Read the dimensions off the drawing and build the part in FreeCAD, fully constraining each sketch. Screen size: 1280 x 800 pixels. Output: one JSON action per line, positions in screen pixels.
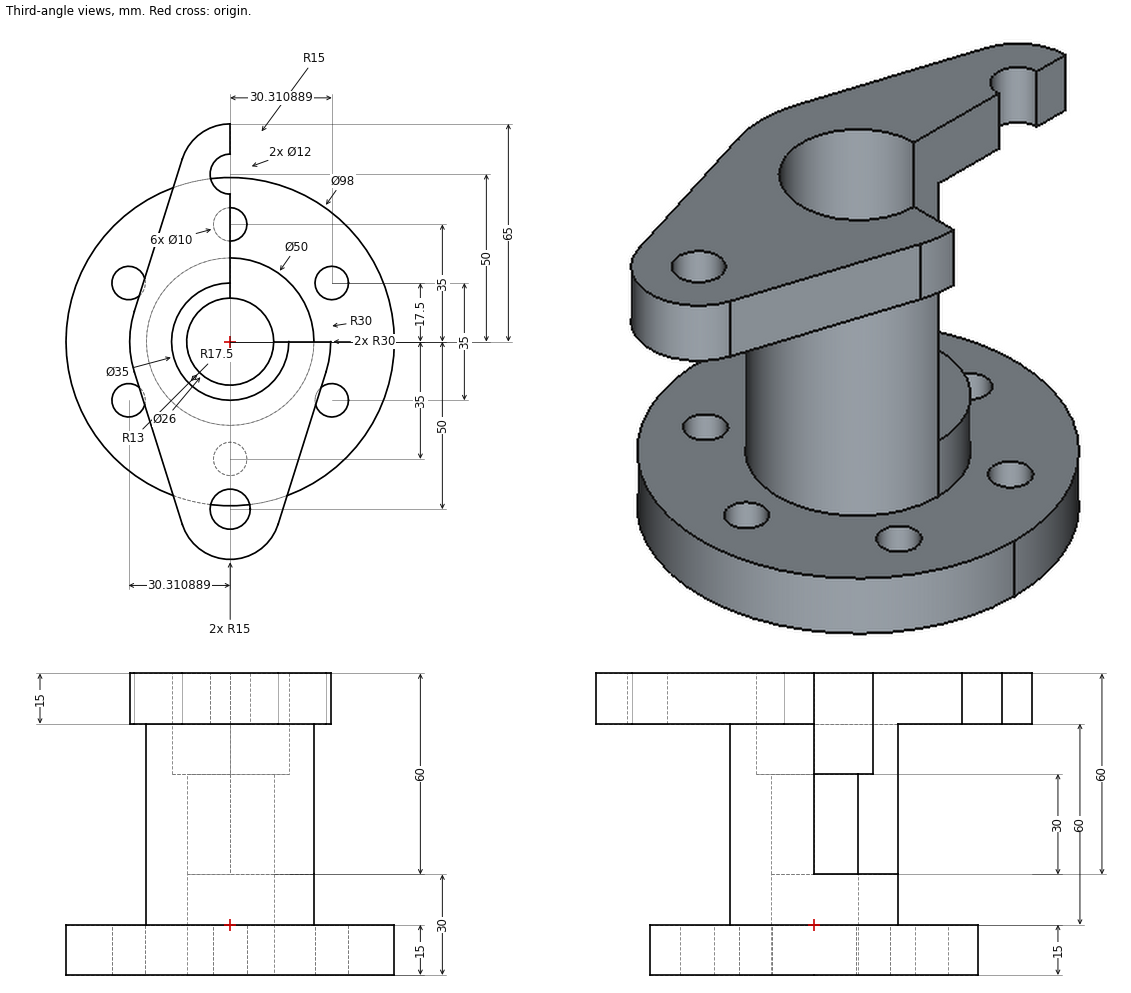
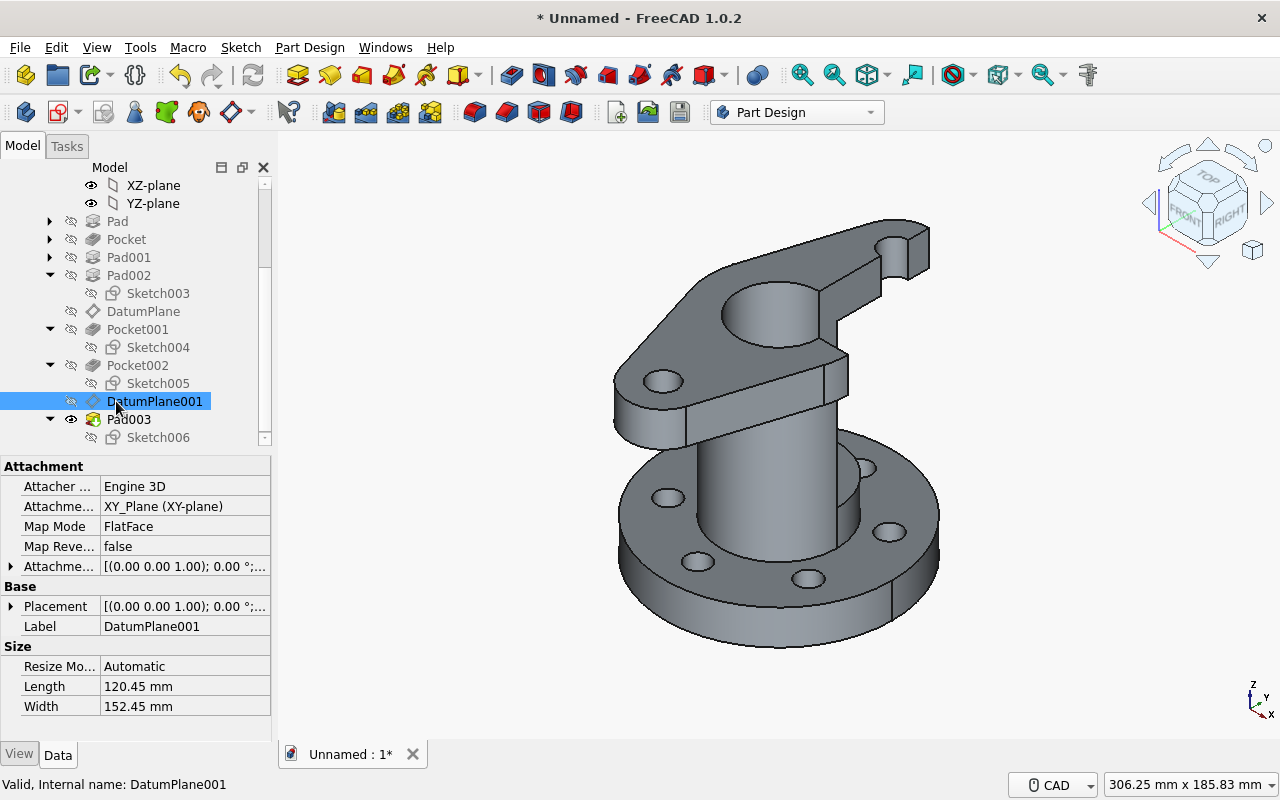
{"action": "key", "text": "2"}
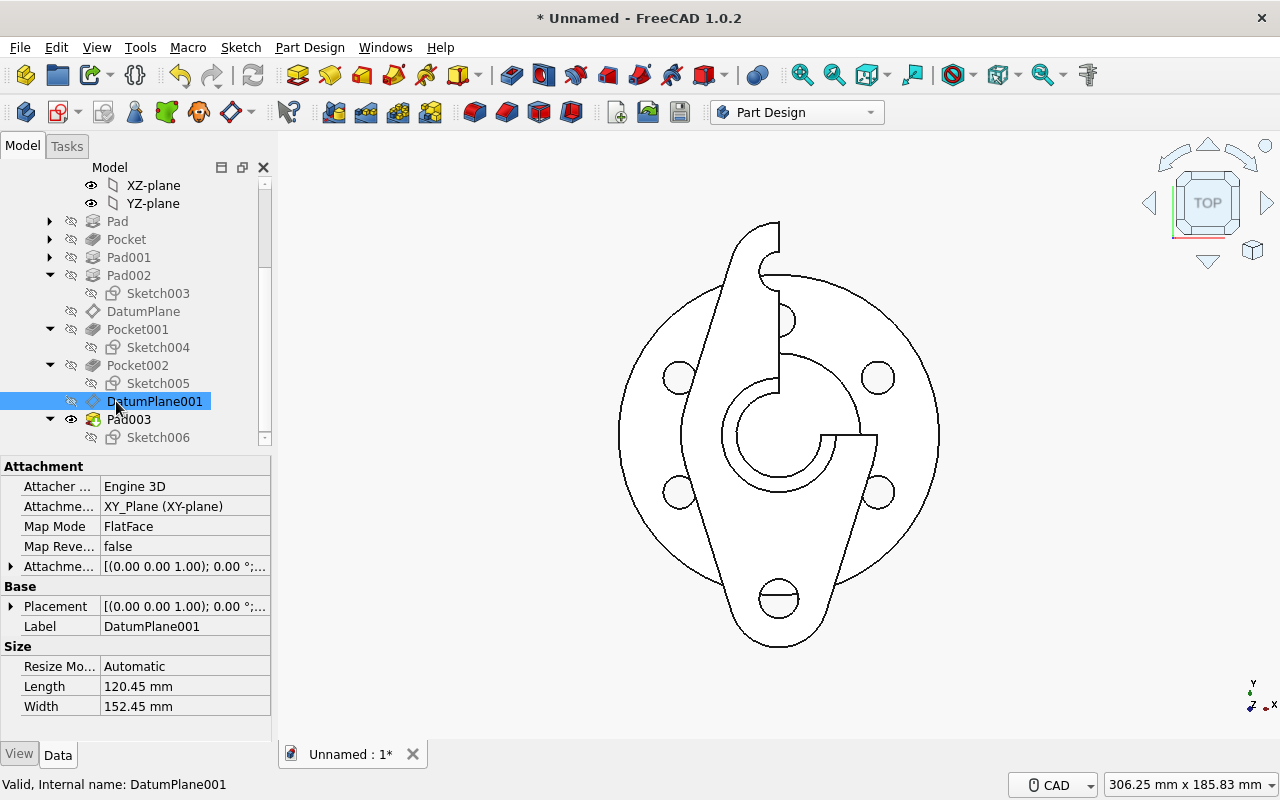
{"action": "left_click", "coordinate": [781, 432]}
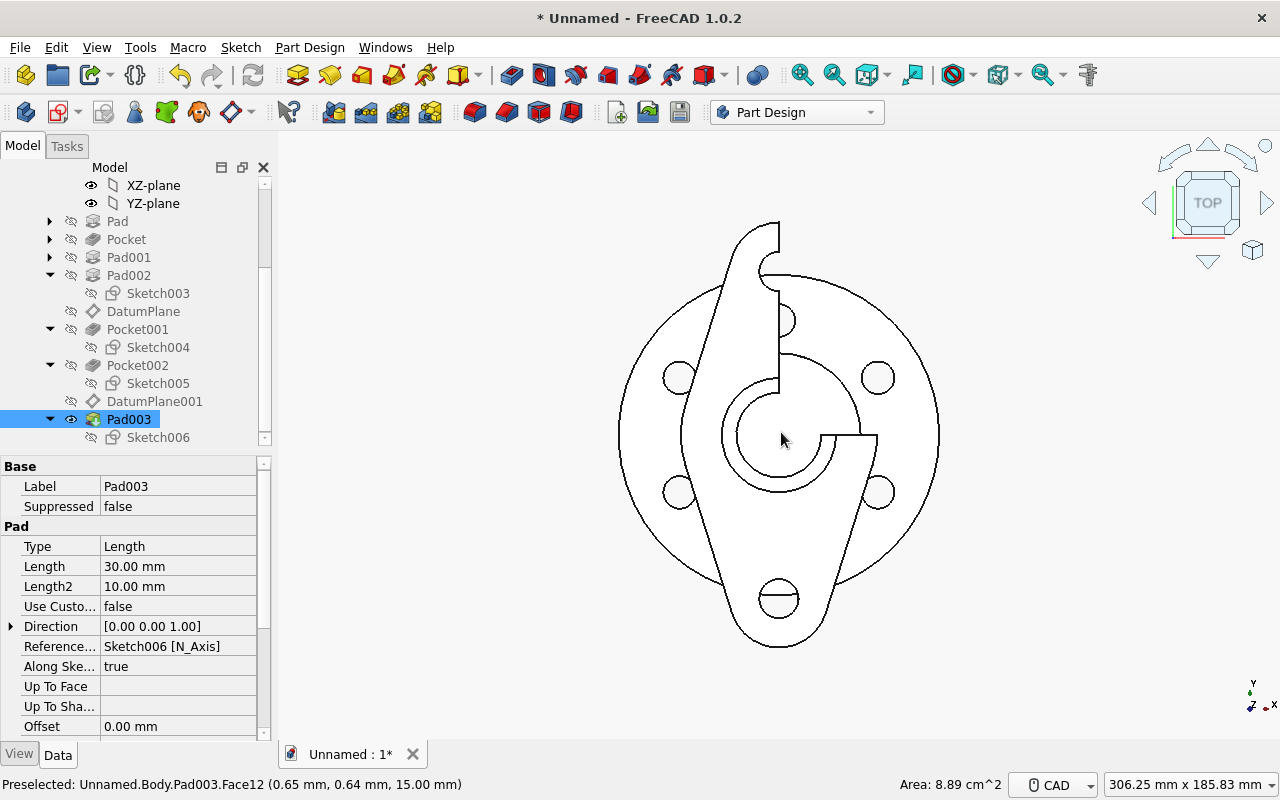
{"action": "left_click", "coordinate": [58, 112]}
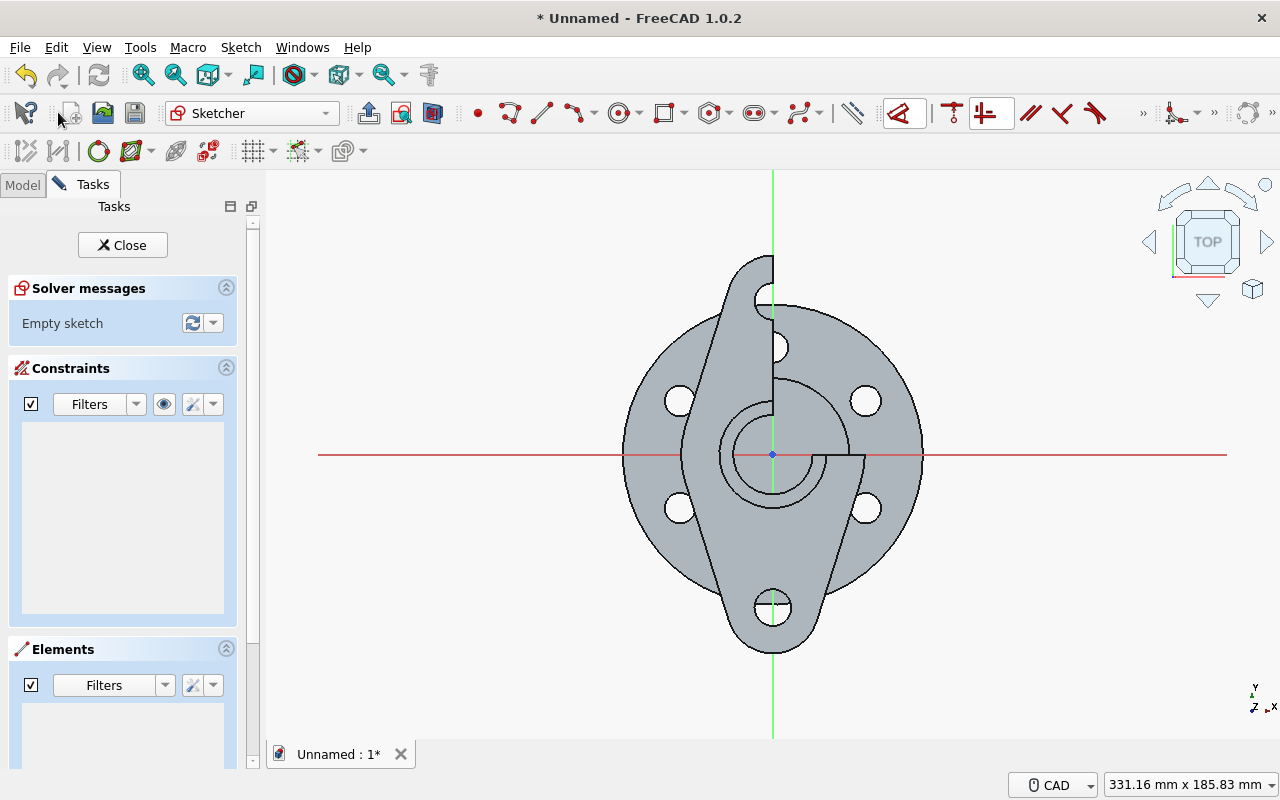
{"action": "left_click", "coordinate": [434, 114]}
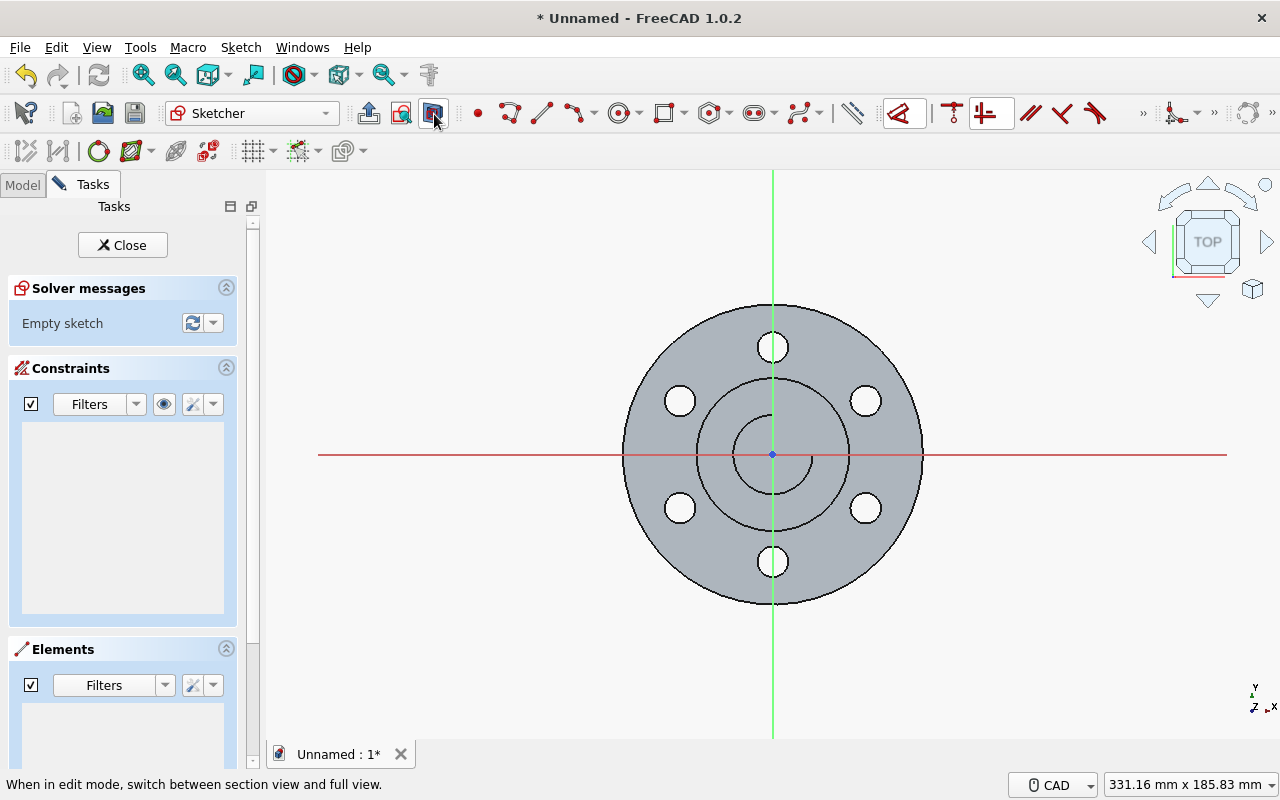
{"action": "scroll", "coordinate": [790, 455], "scroll_direction": "up", "scroll_amount": 8}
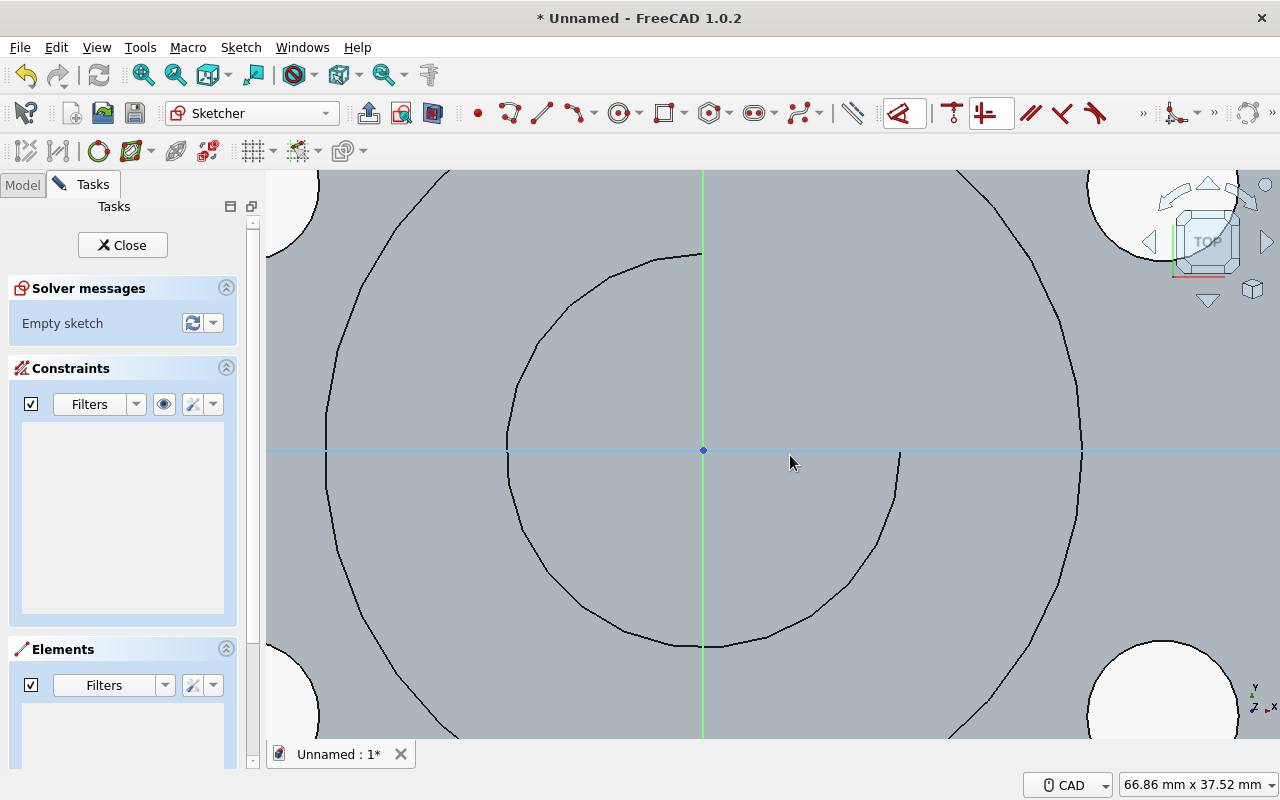
{"action": "left_click", "coordinate": [620, 114]}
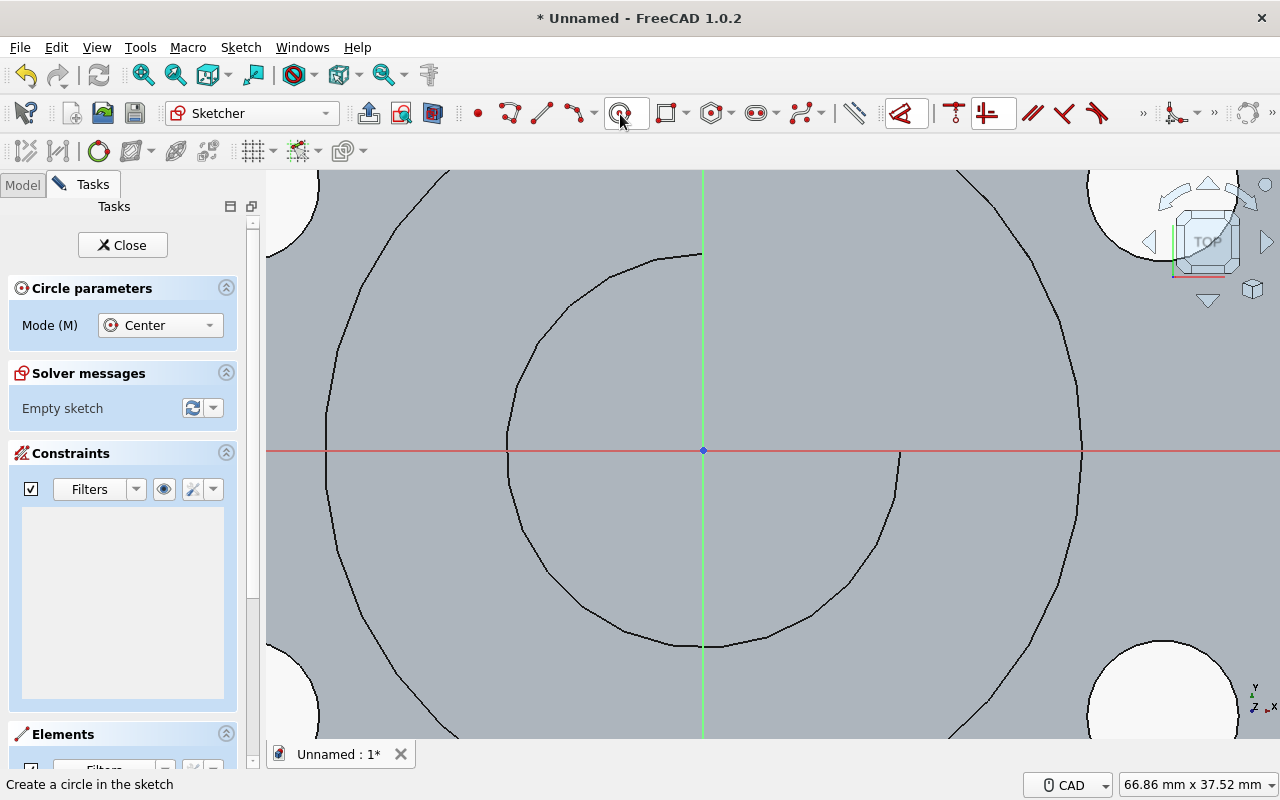
{"action": "left_click", "coordinate": [703, 451]}
{"action": "left_click", "coordinate": [843, 312]}
{"action": "key", "text": "Escape"}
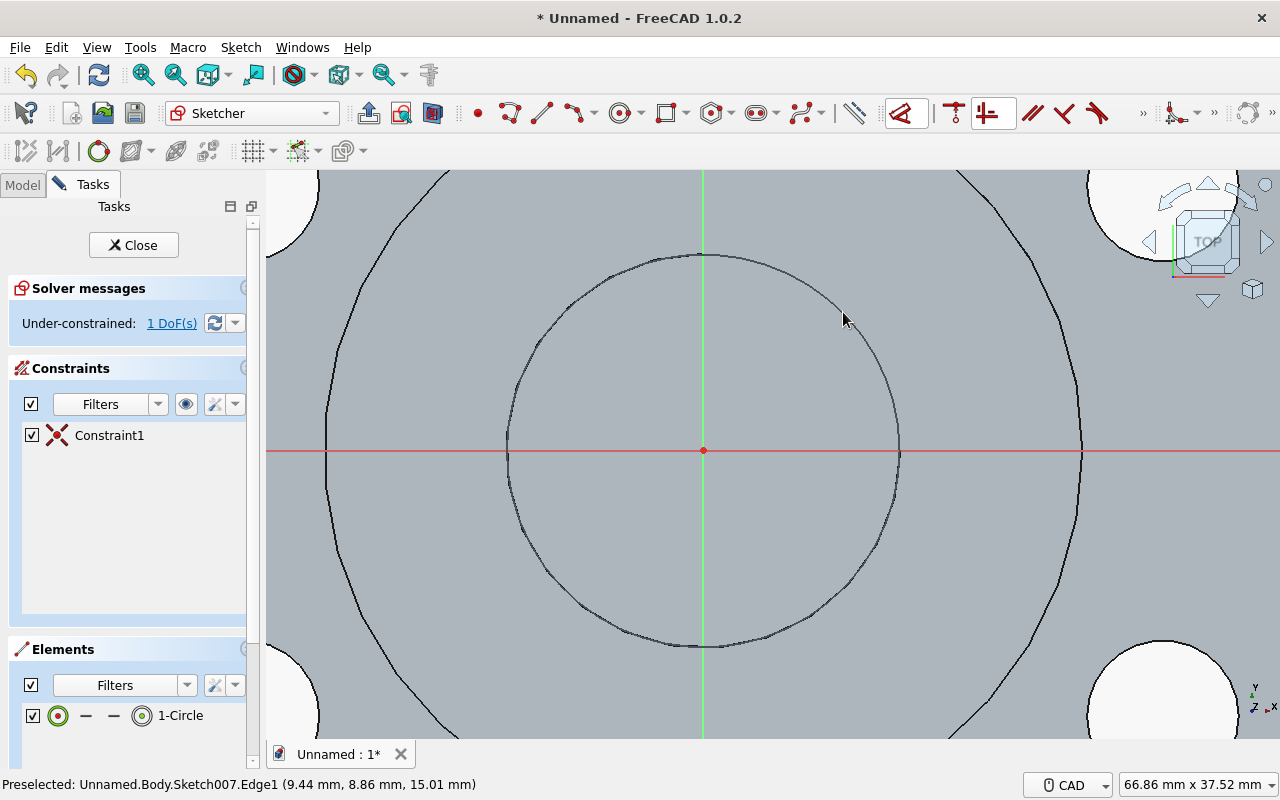
{"action": "left_click", "coordinate": [842, 312]}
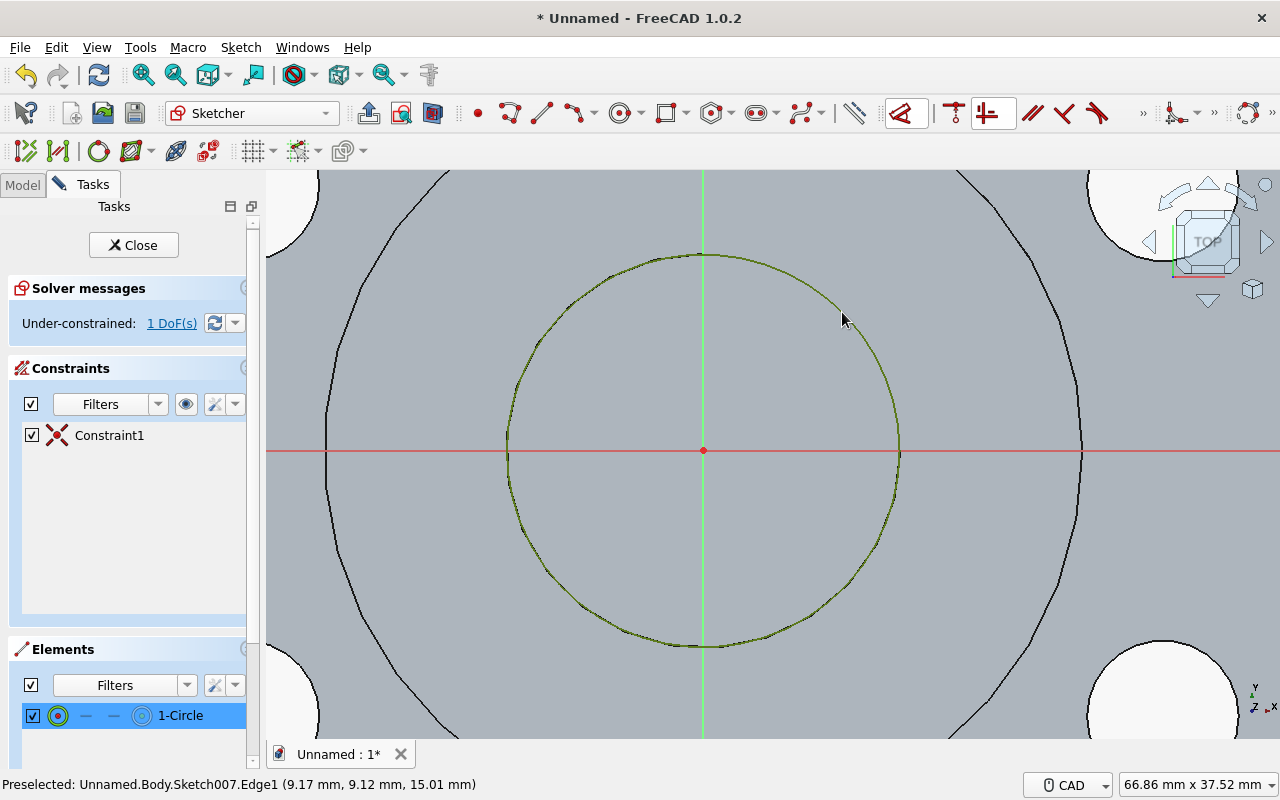
{"action": "left_click", "coordinate": [922, 114]}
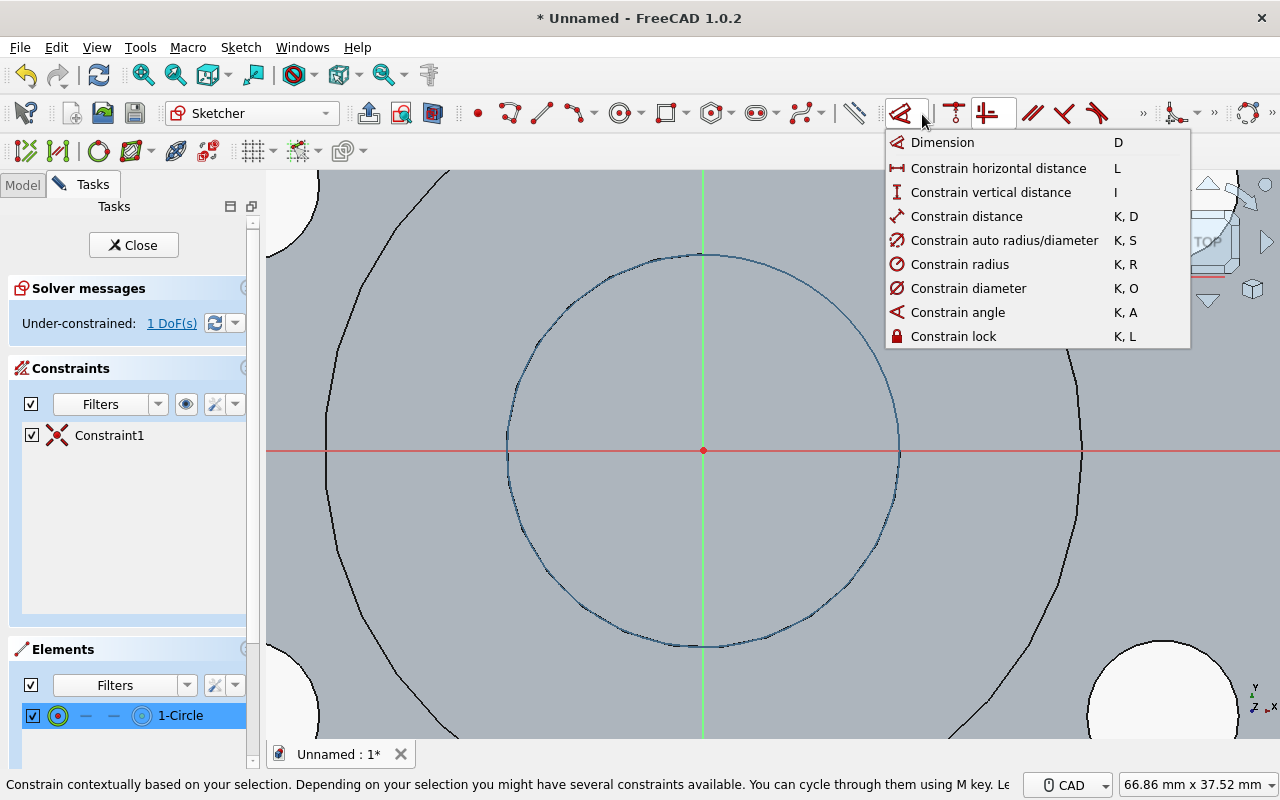
{"action": "left_click", "coordinate": [1038, 288]}